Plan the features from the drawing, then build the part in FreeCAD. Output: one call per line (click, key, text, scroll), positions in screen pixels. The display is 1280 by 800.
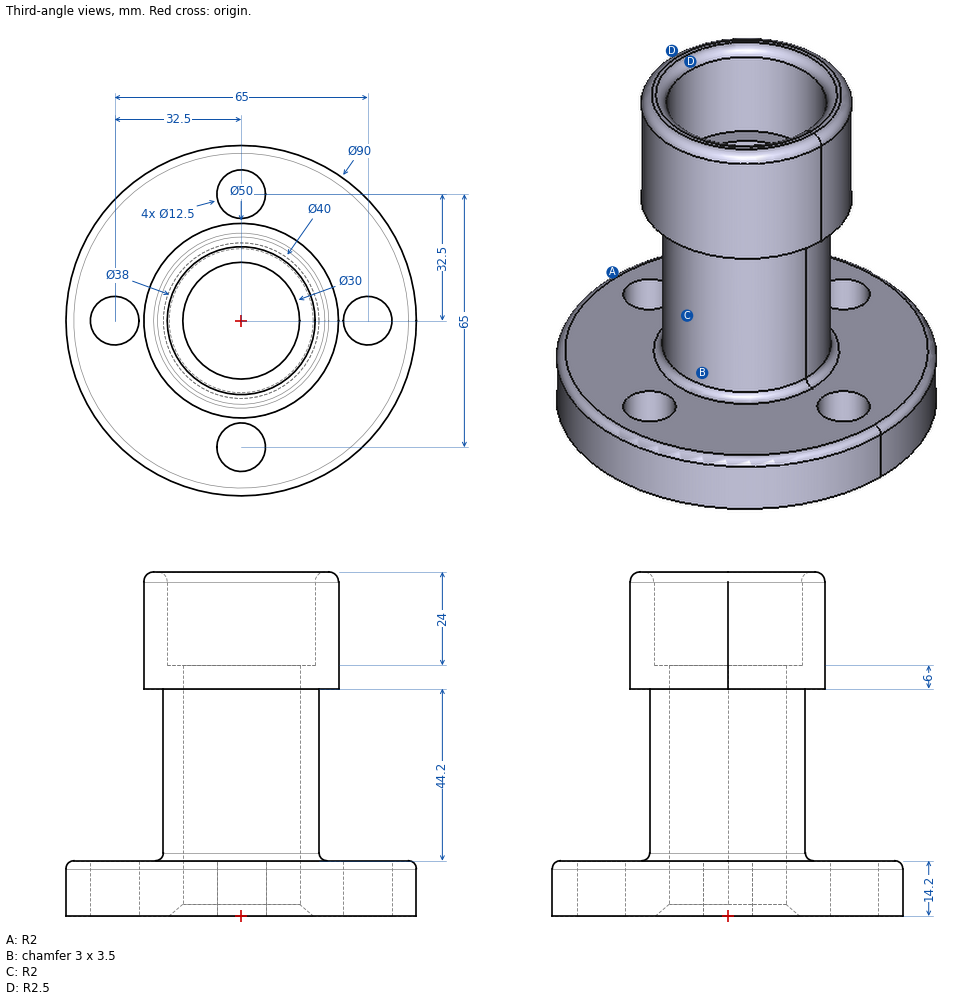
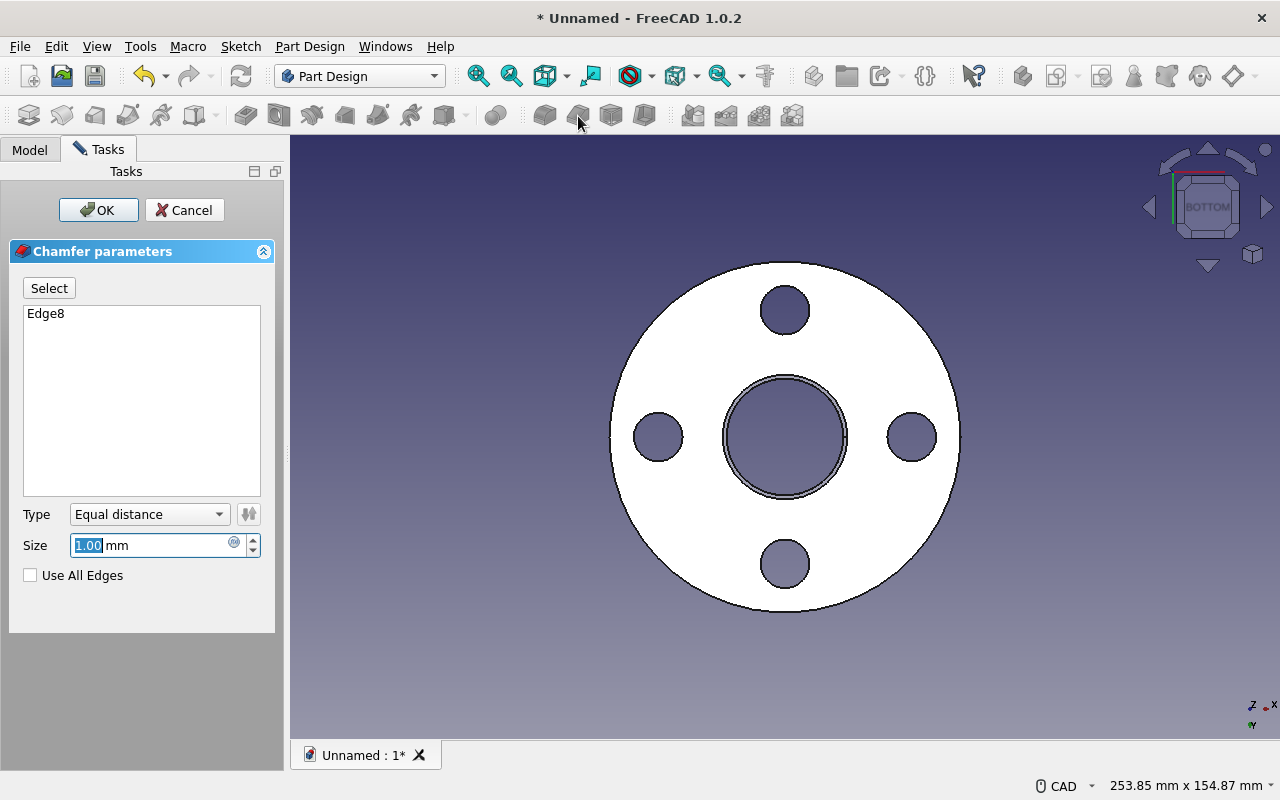
text(3)
key(Tab)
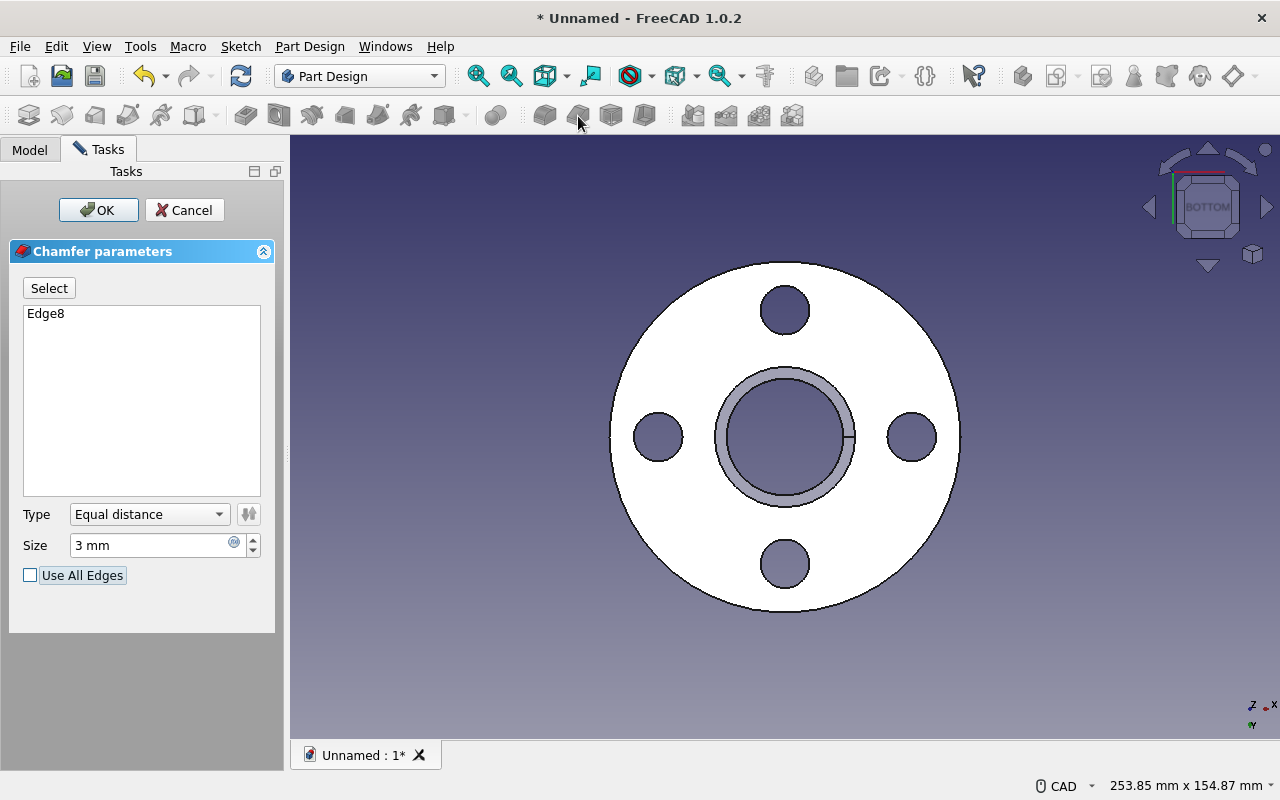
click(150, 514)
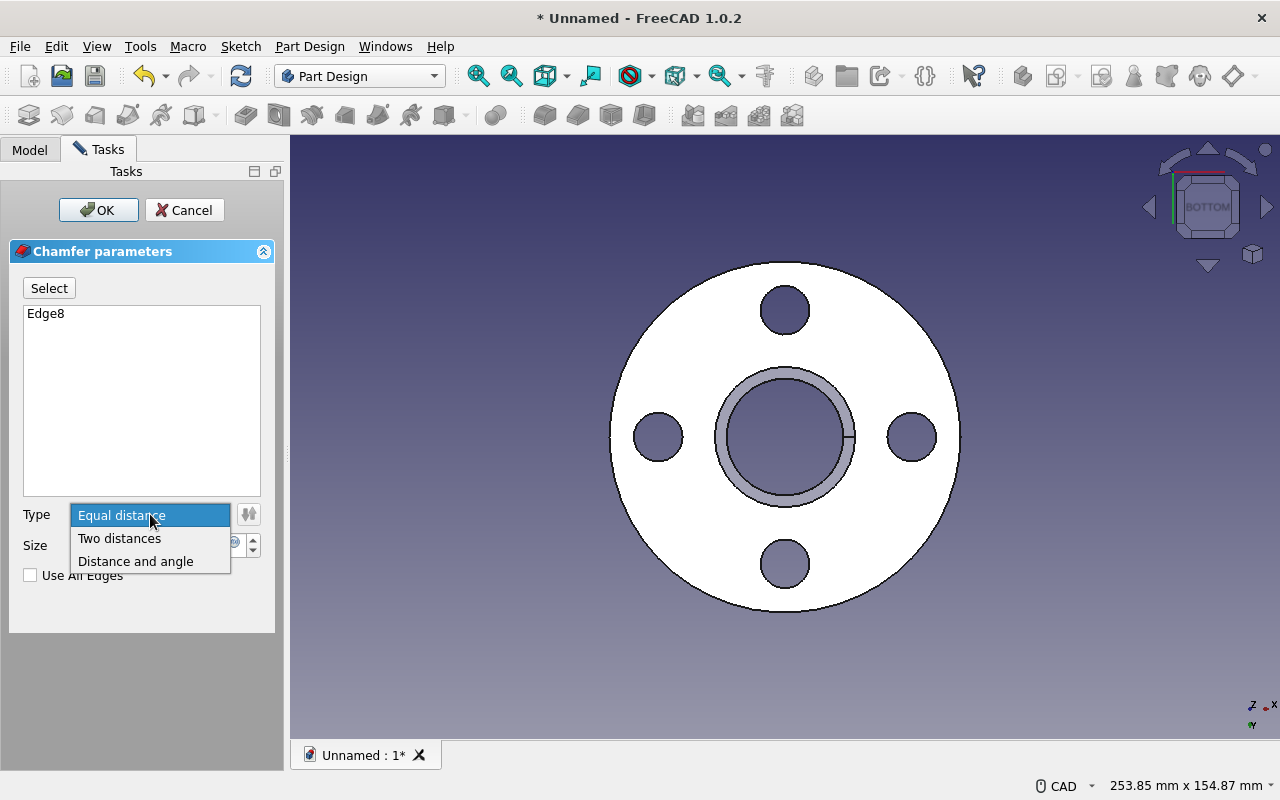
click(148, 538)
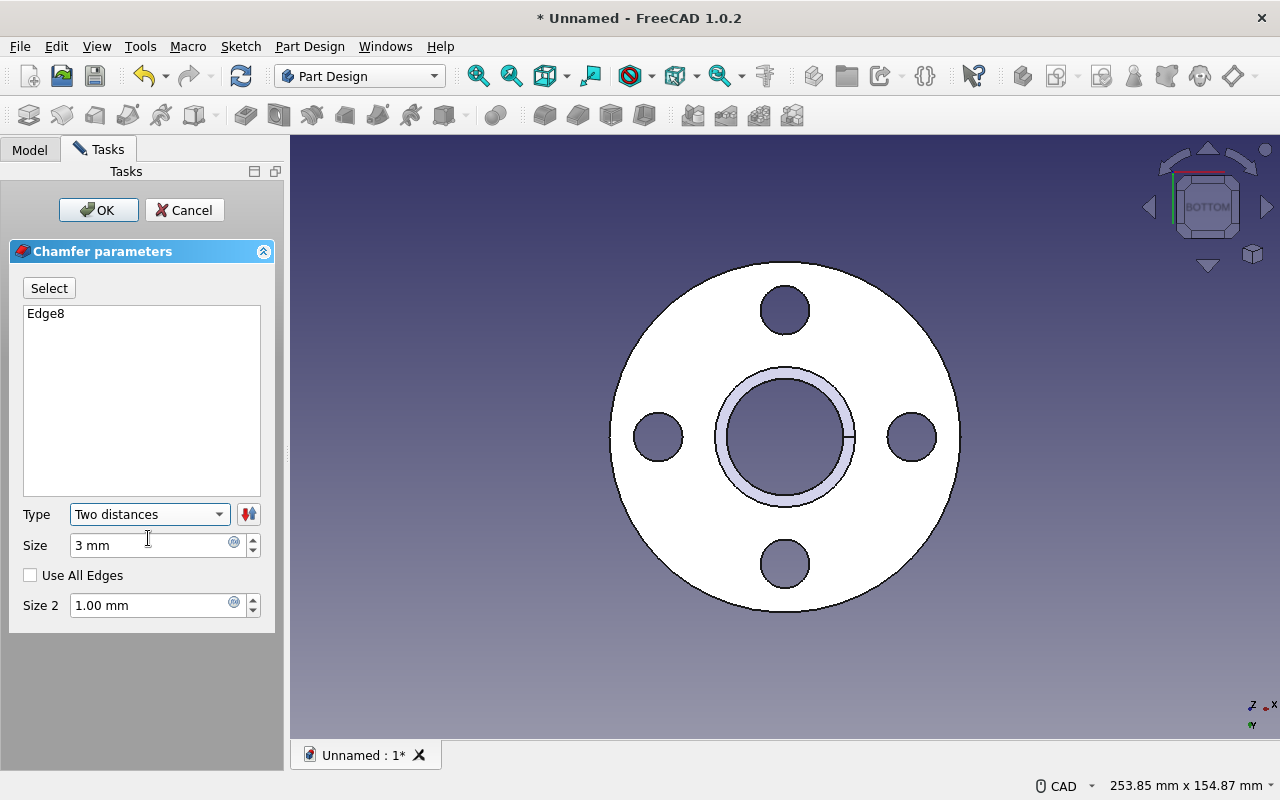
triple_click(158, 606)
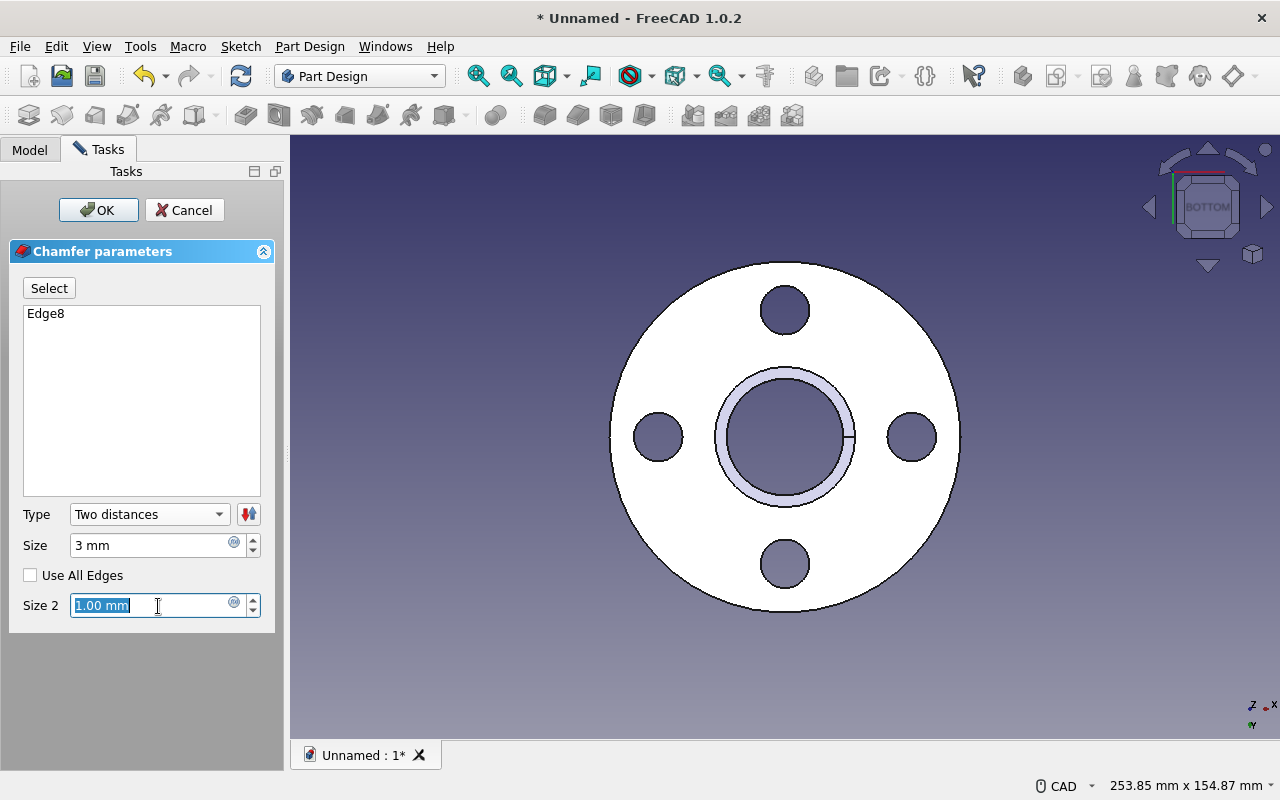
text(3.5)
key(Tab)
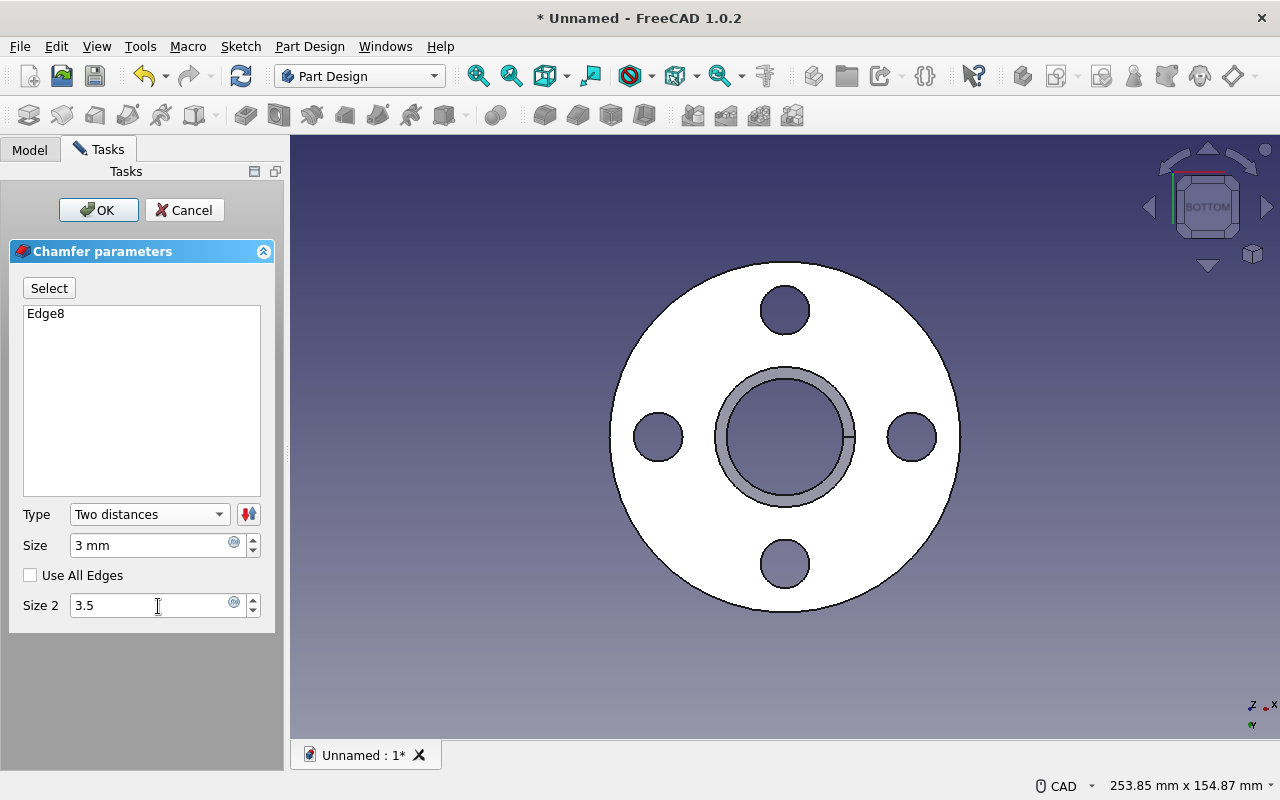
click(249, 514)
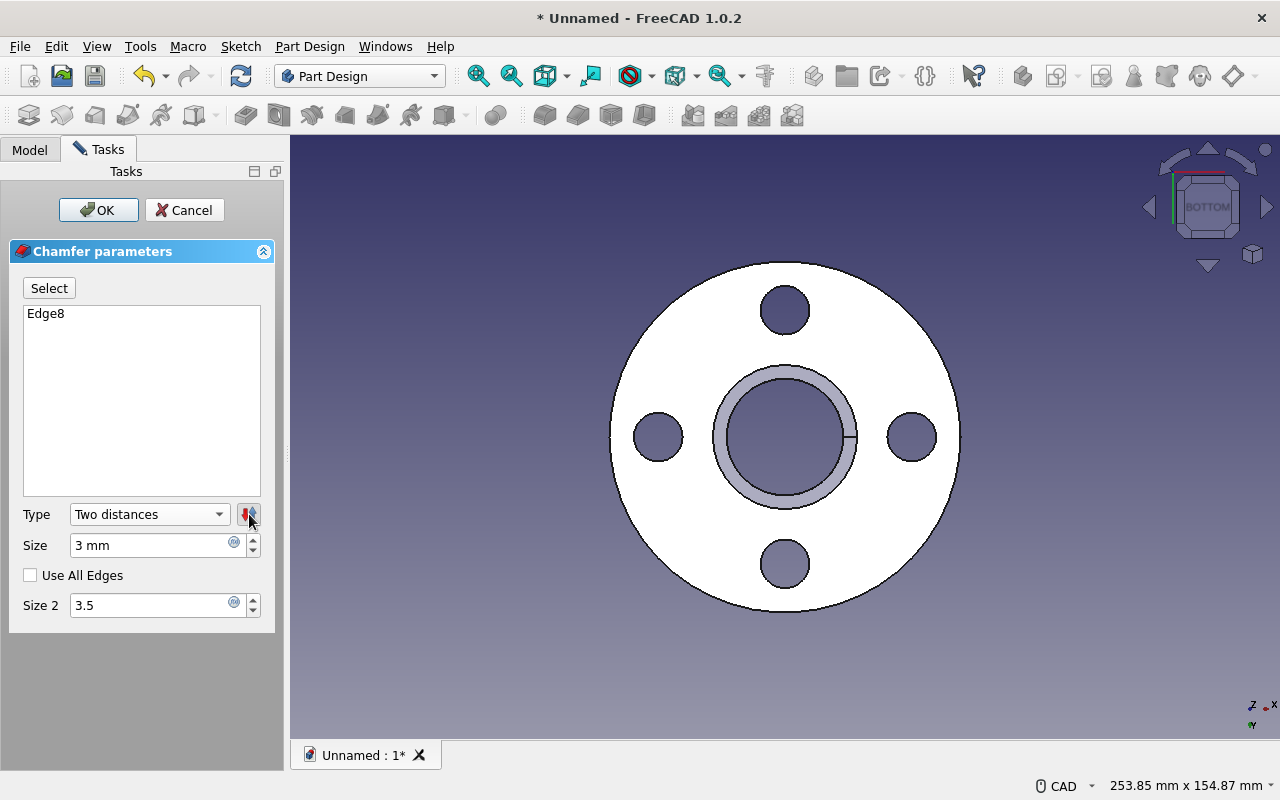
click(99, 210)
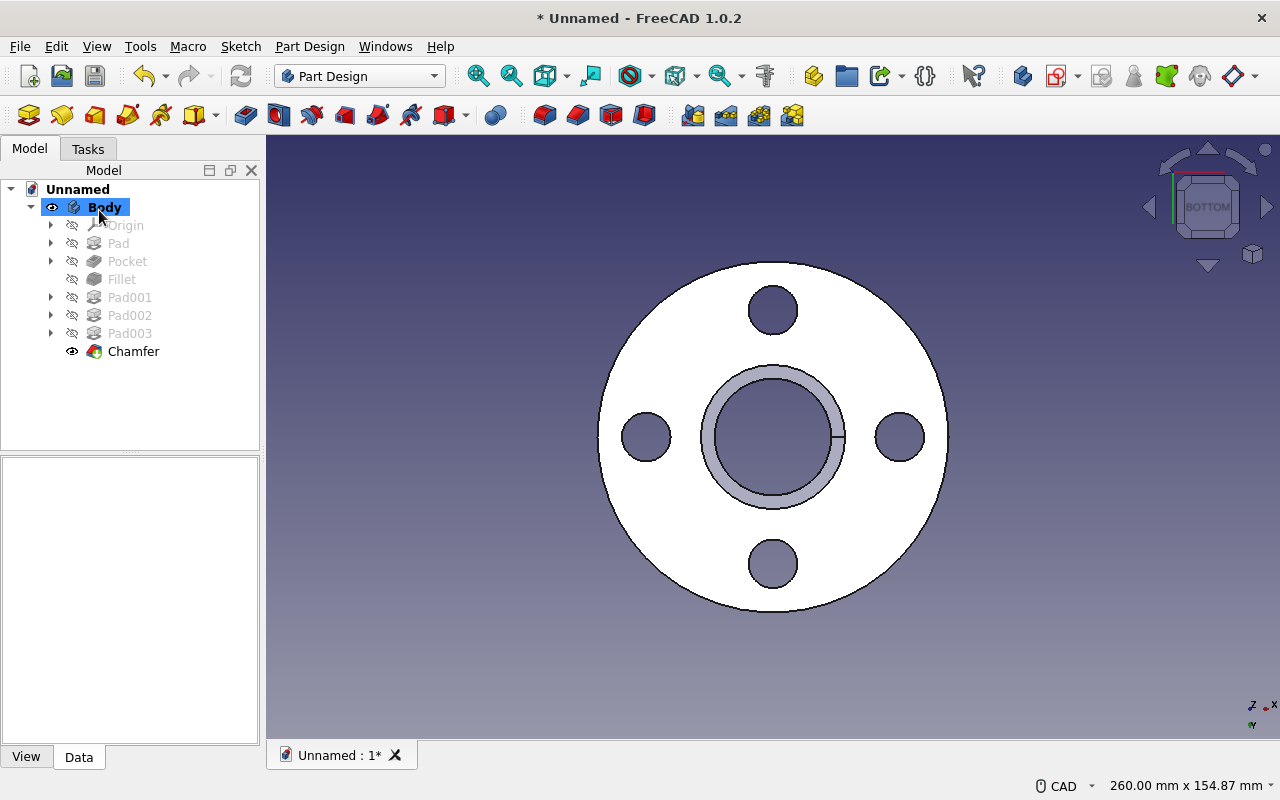
key(0)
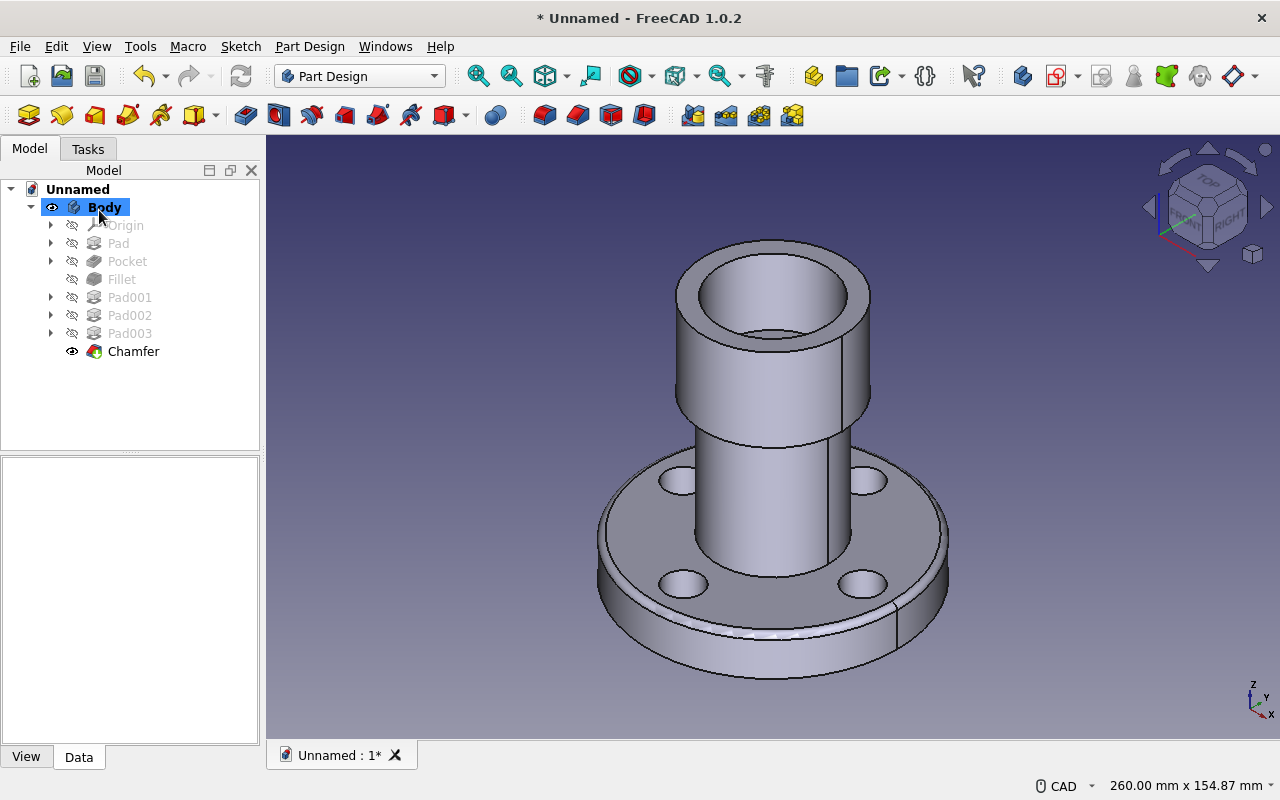
key(2)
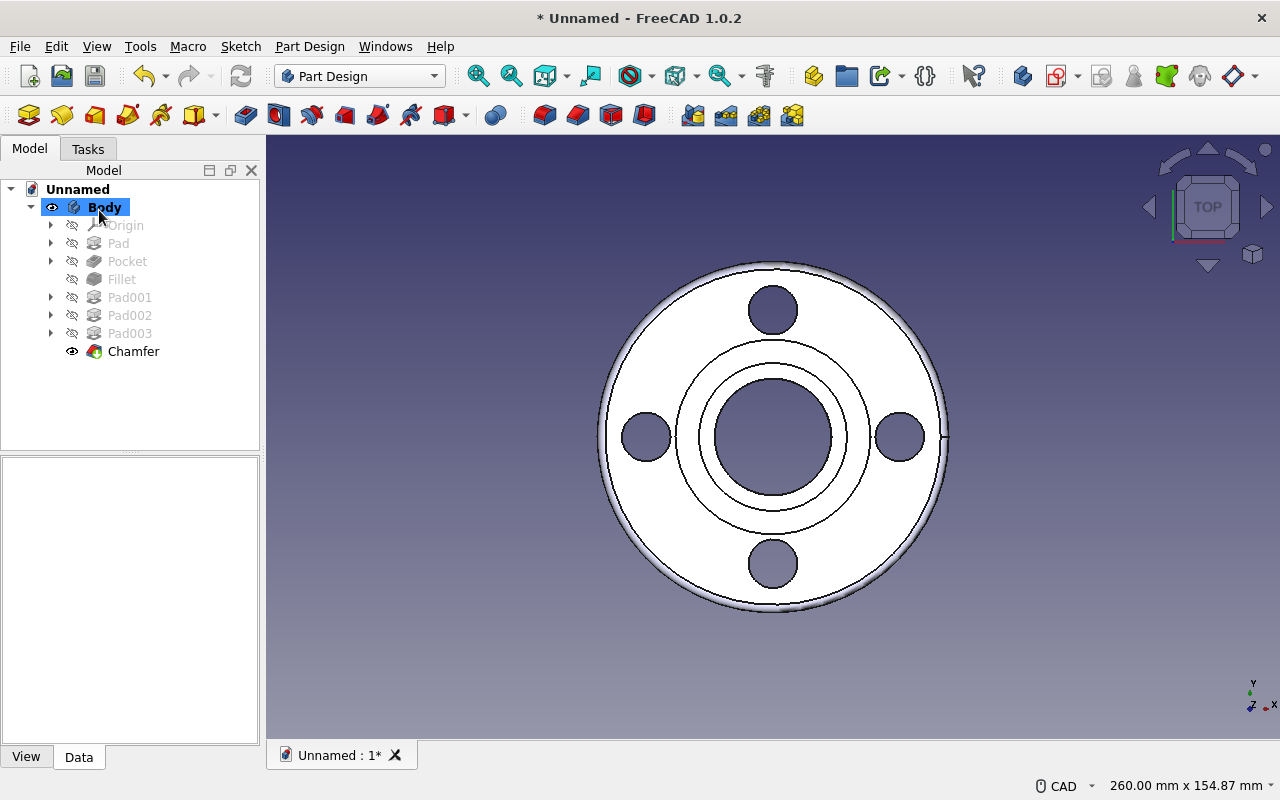
key(1)